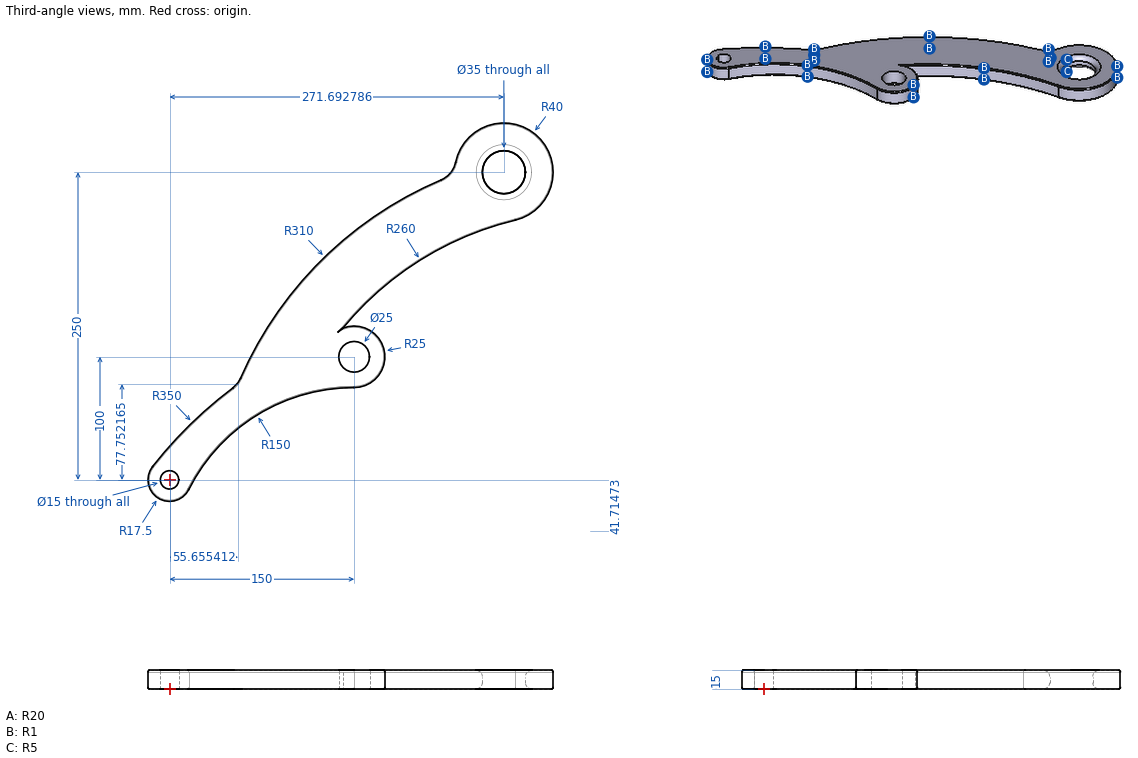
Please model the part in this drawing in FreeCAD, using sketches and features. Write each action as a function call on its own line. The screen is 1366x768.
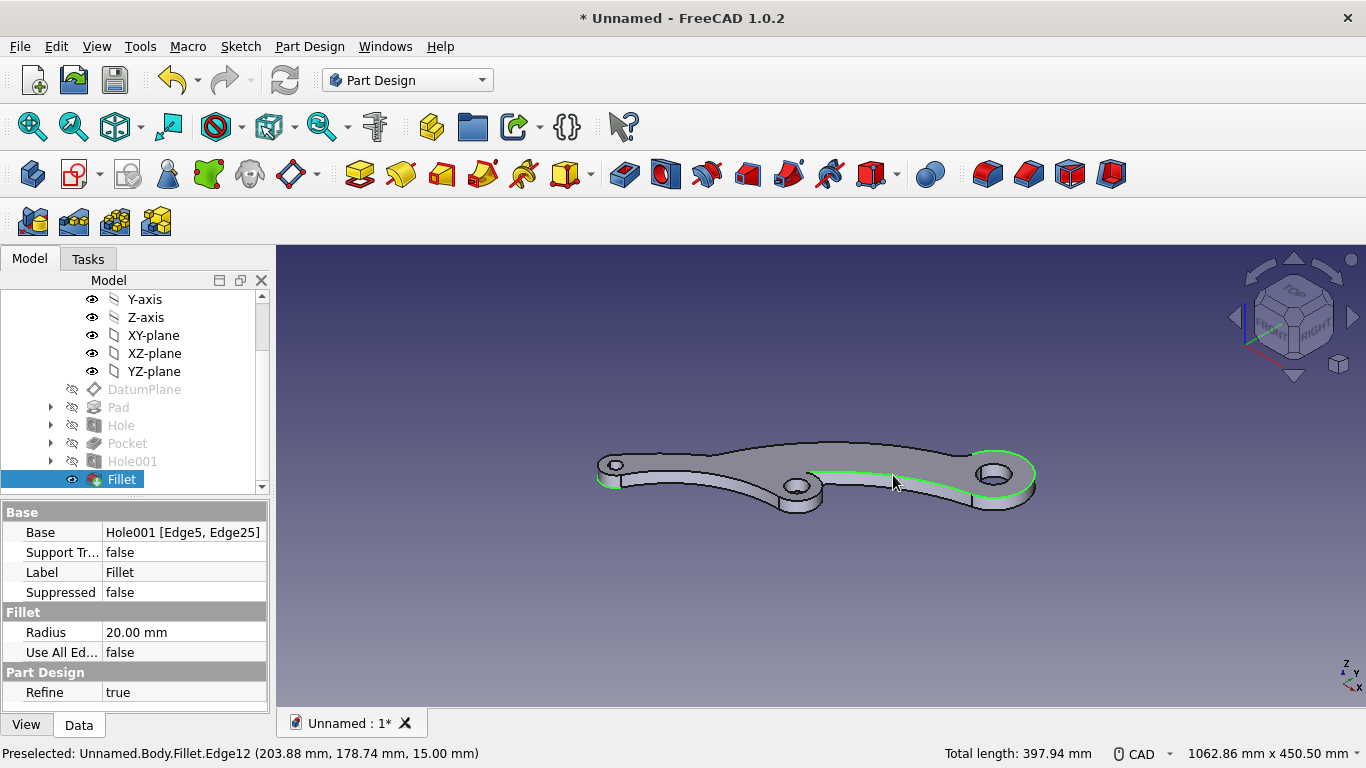
click(818, 493, ctrl)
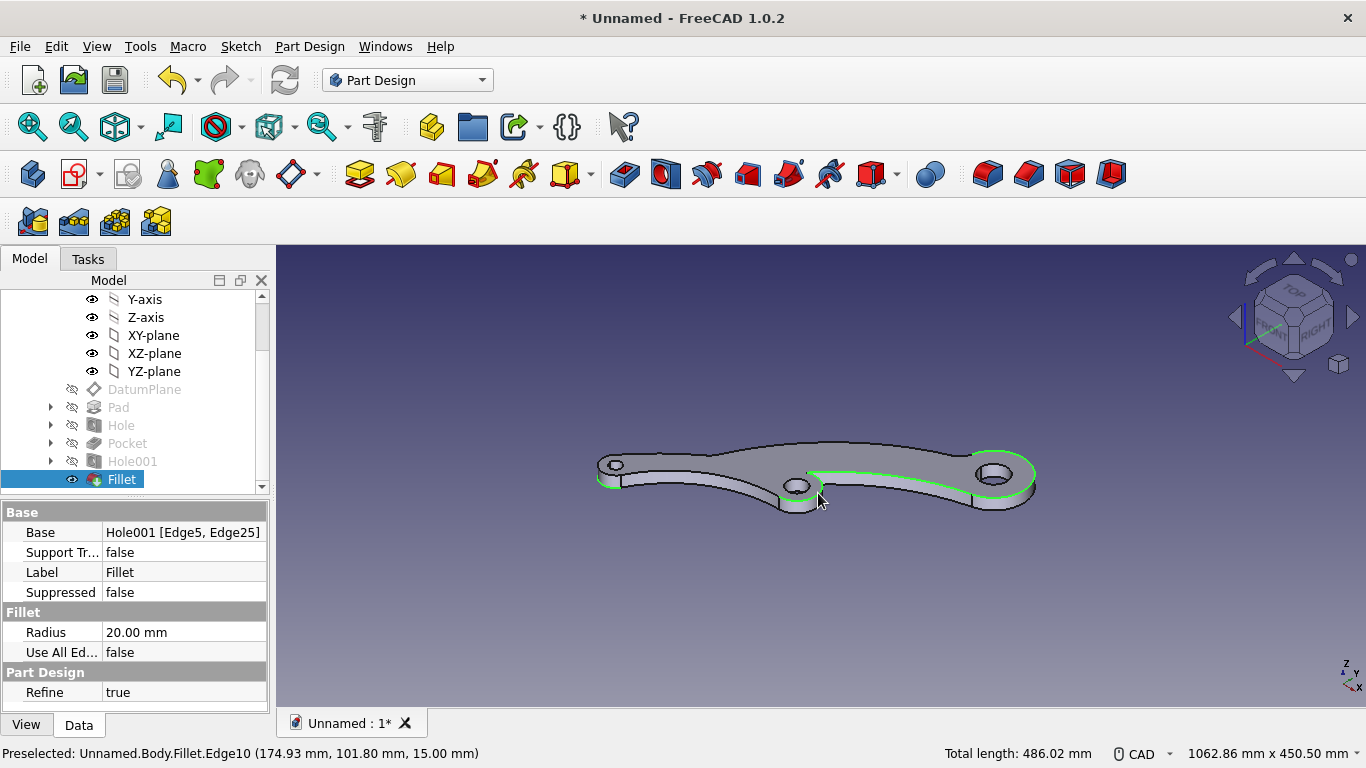
click(705, 472, ctrl)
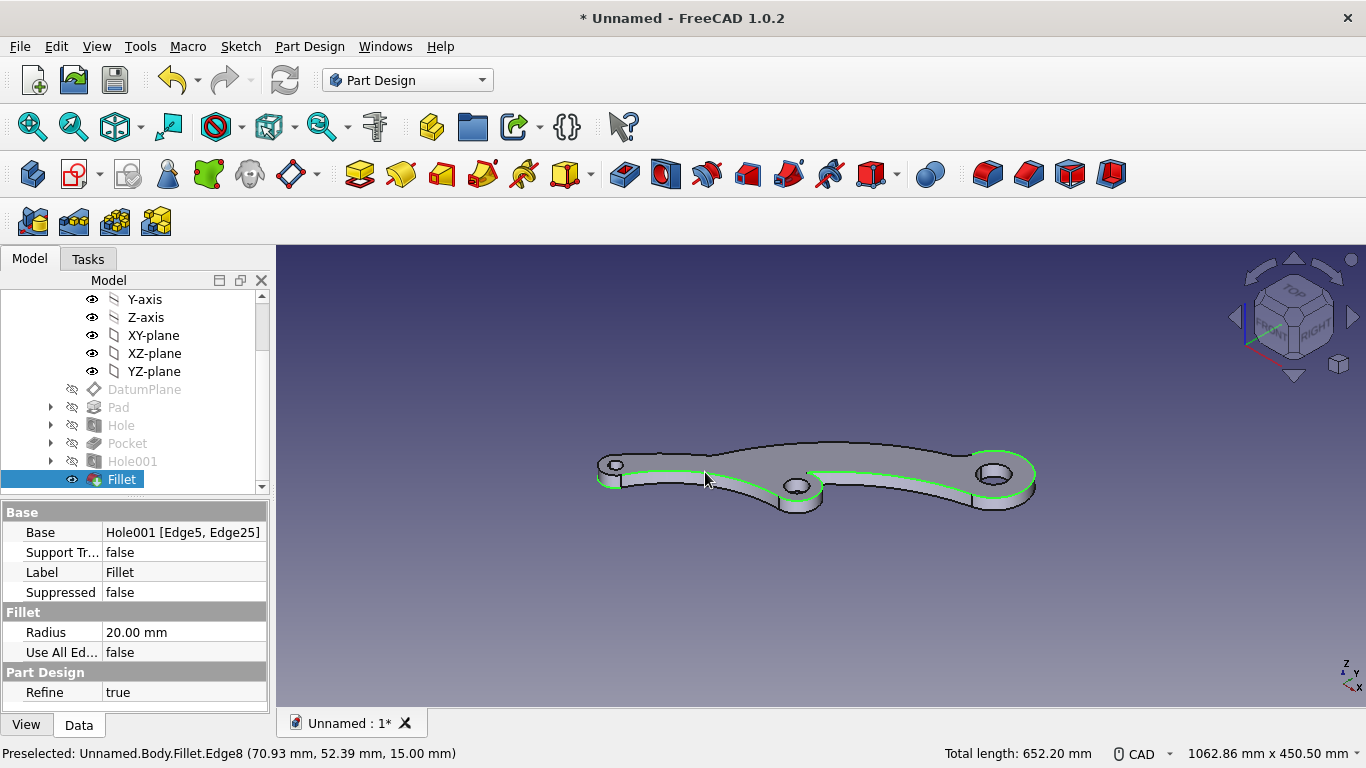
click(598, 466, ctrl)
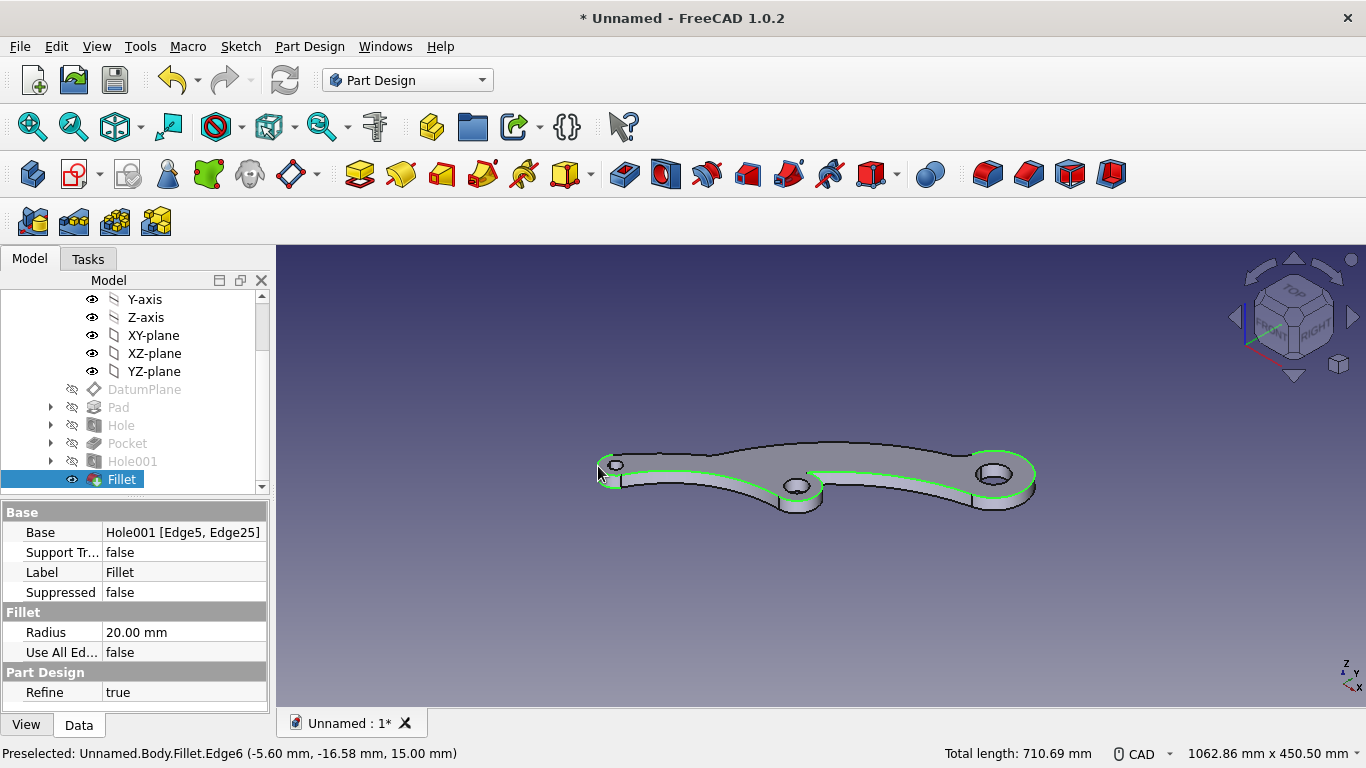
key(2)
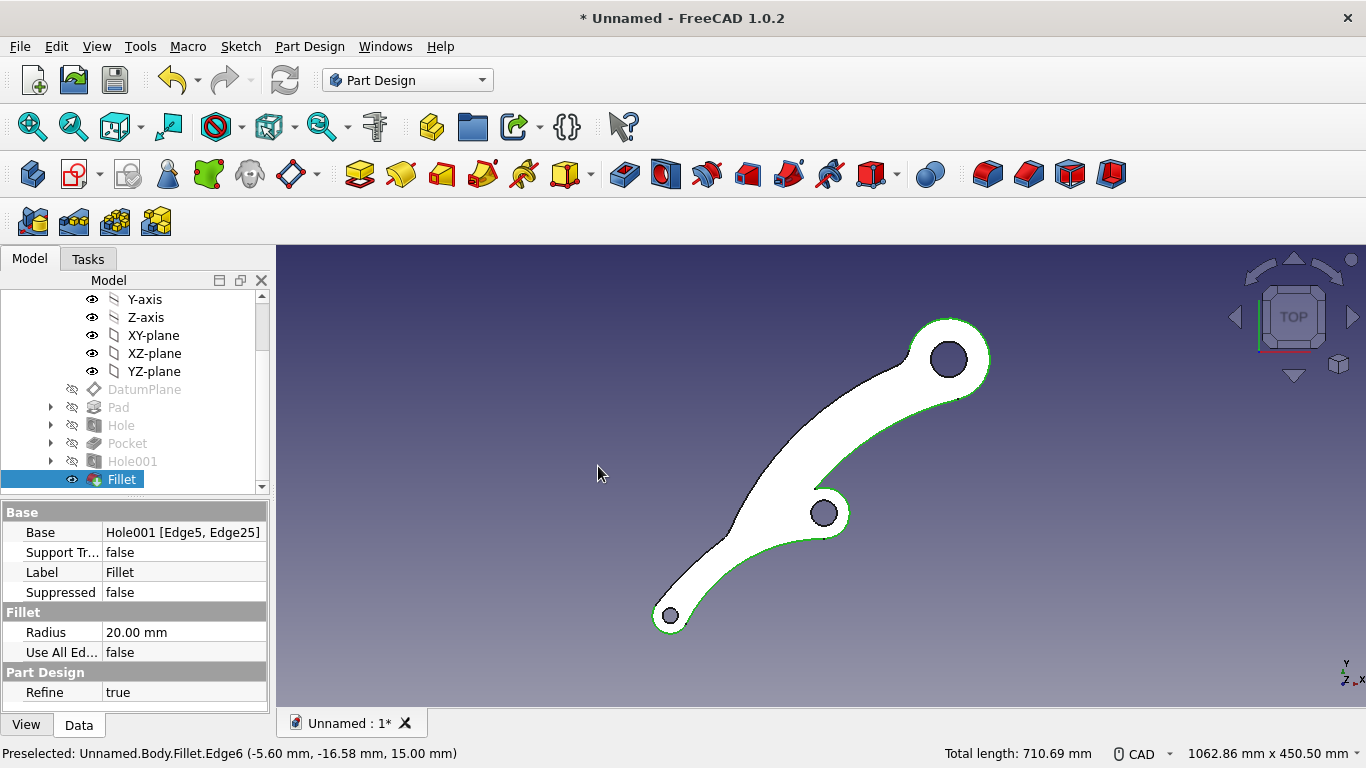
click(797, 431, ctrl)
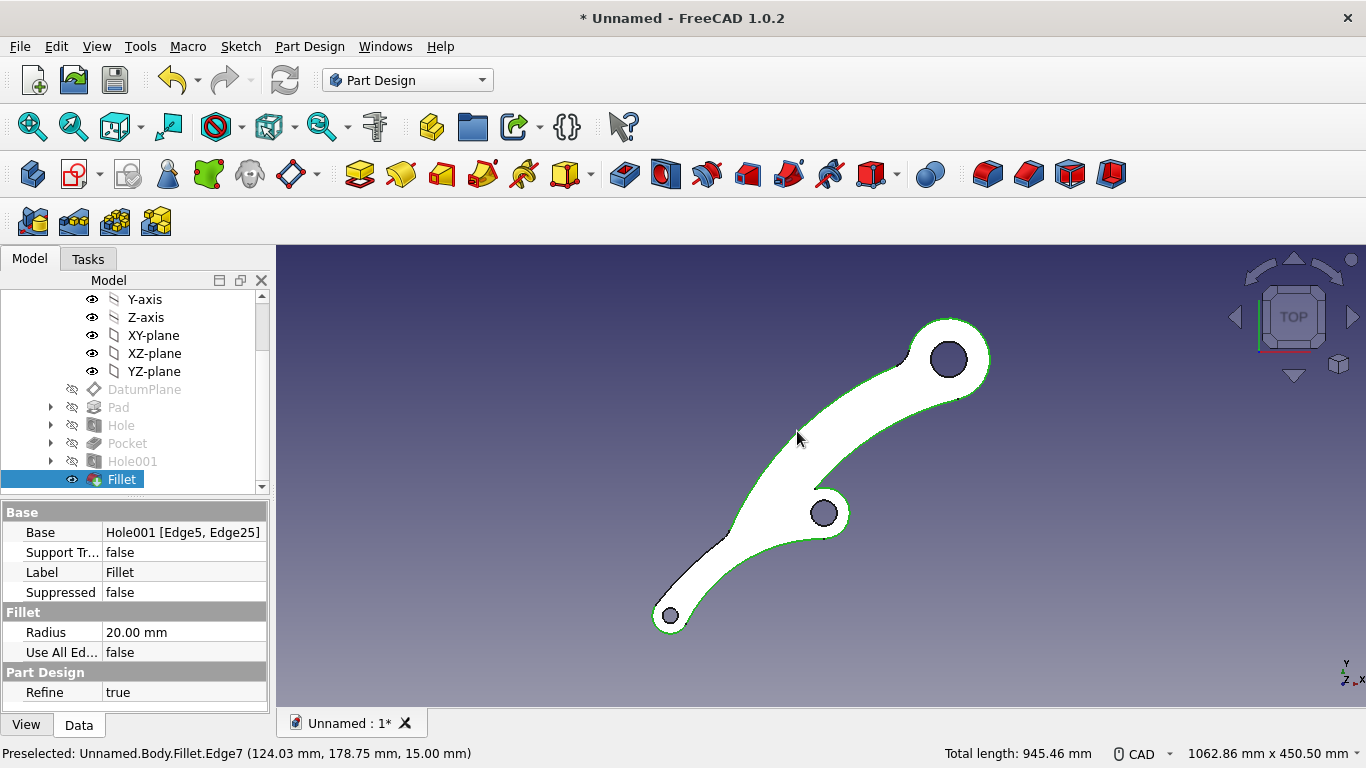
click(687, 569, ctrl)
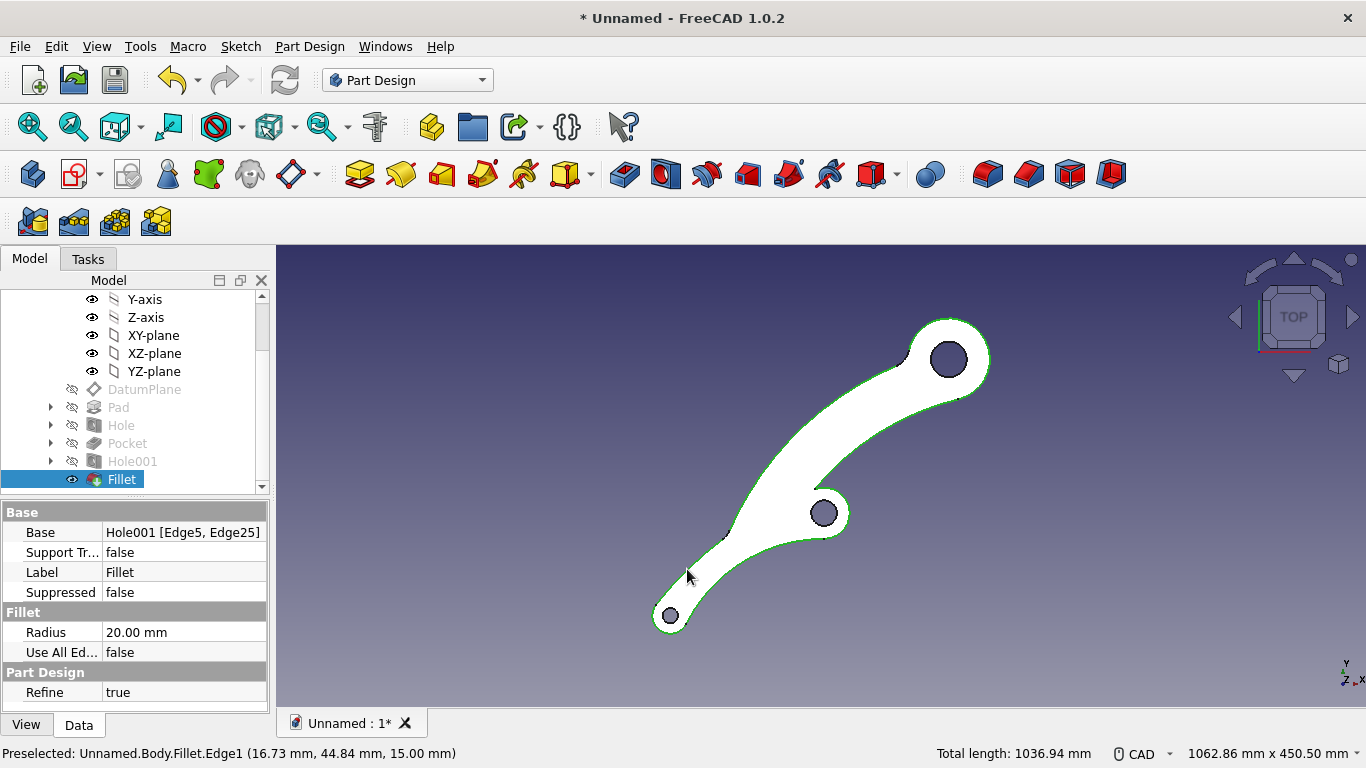
click(904, 359, ctrl)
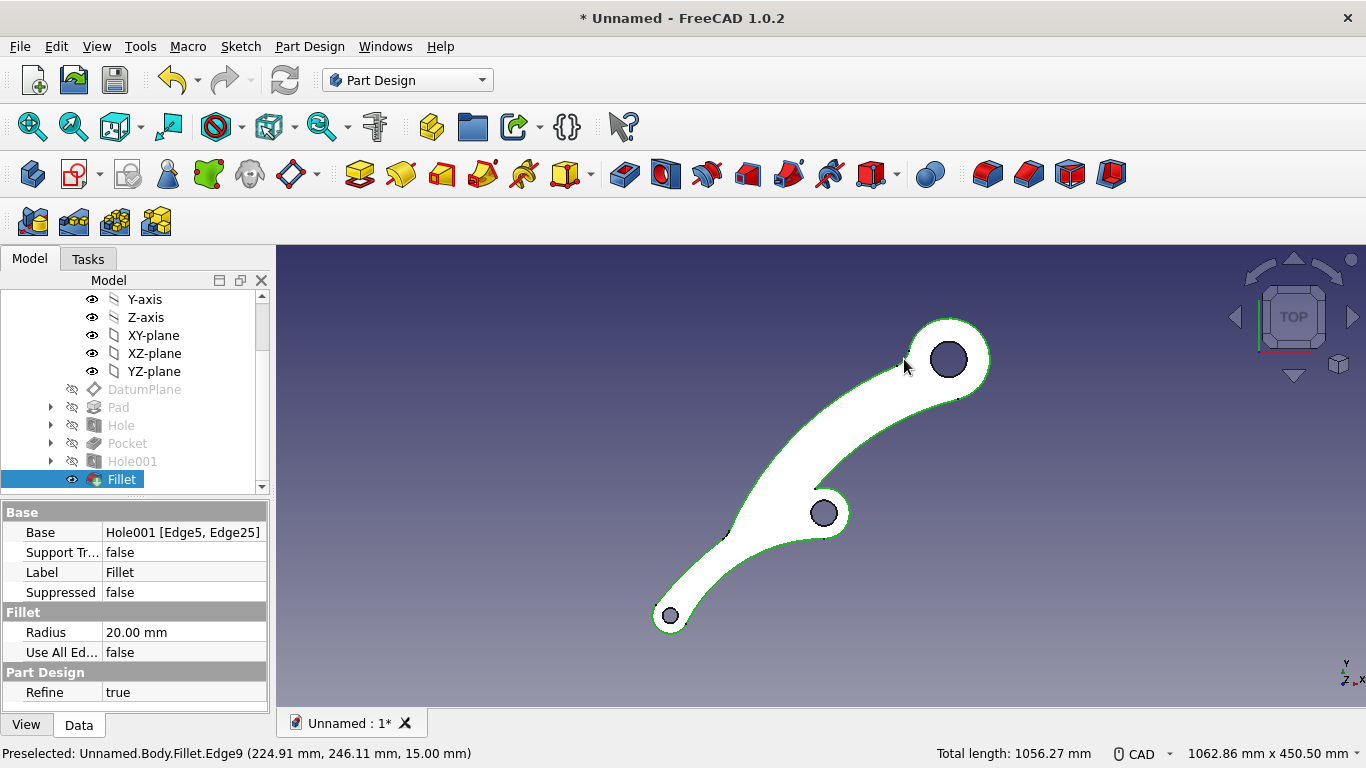
key(0)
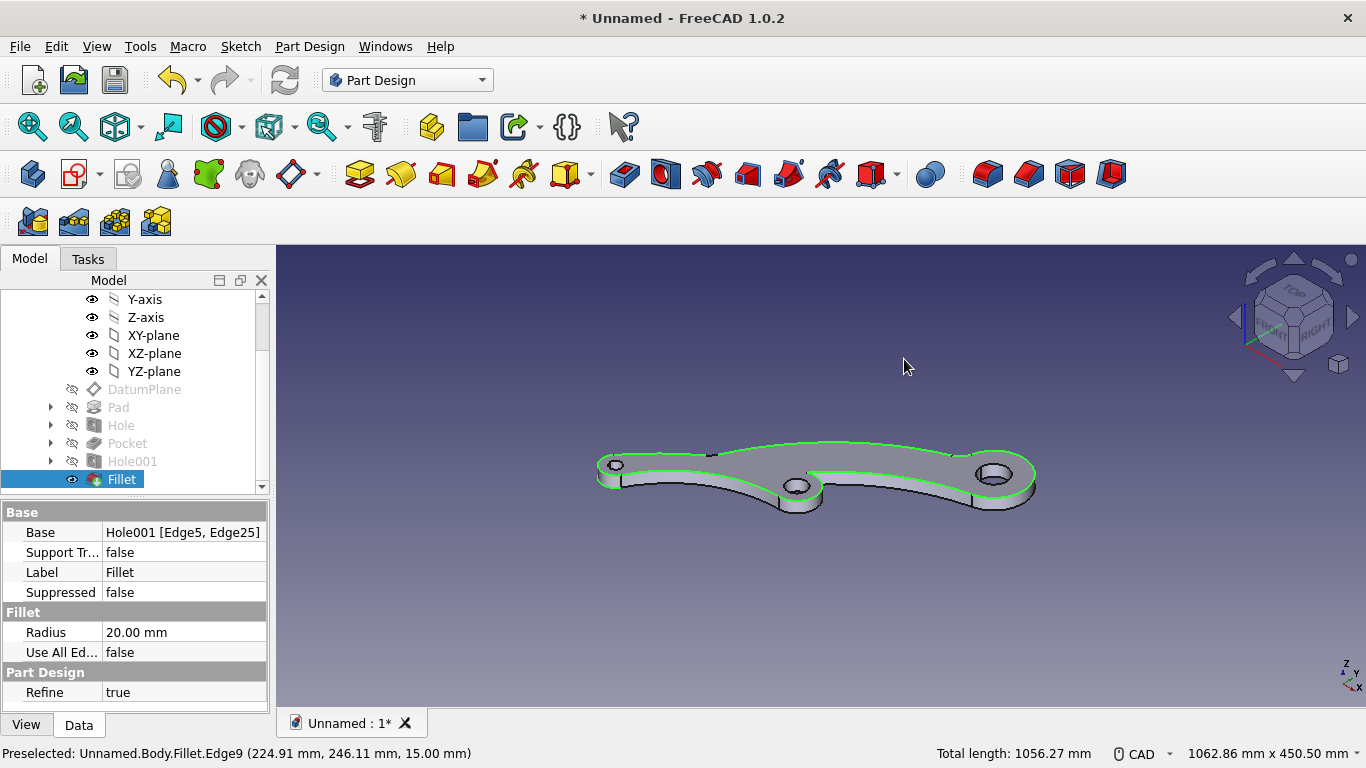
key(1)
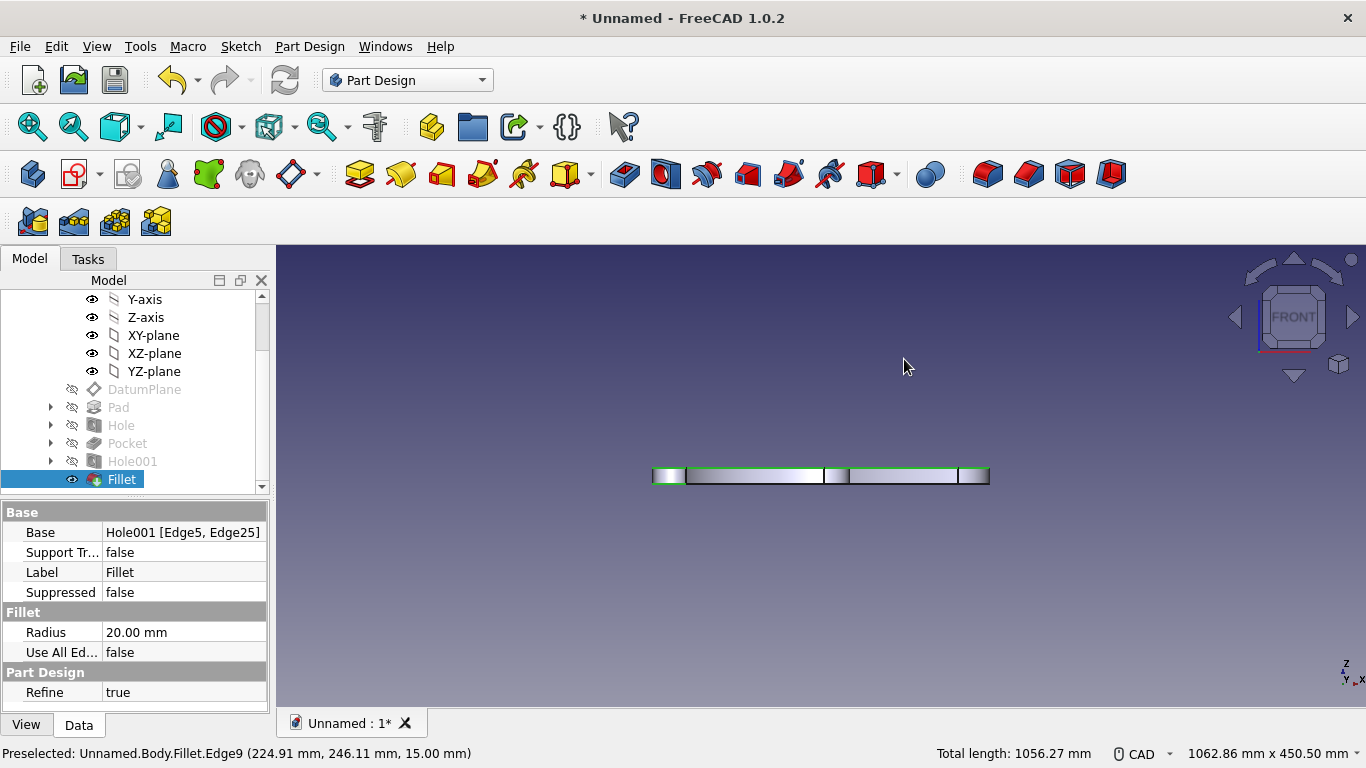
click(33, 128)